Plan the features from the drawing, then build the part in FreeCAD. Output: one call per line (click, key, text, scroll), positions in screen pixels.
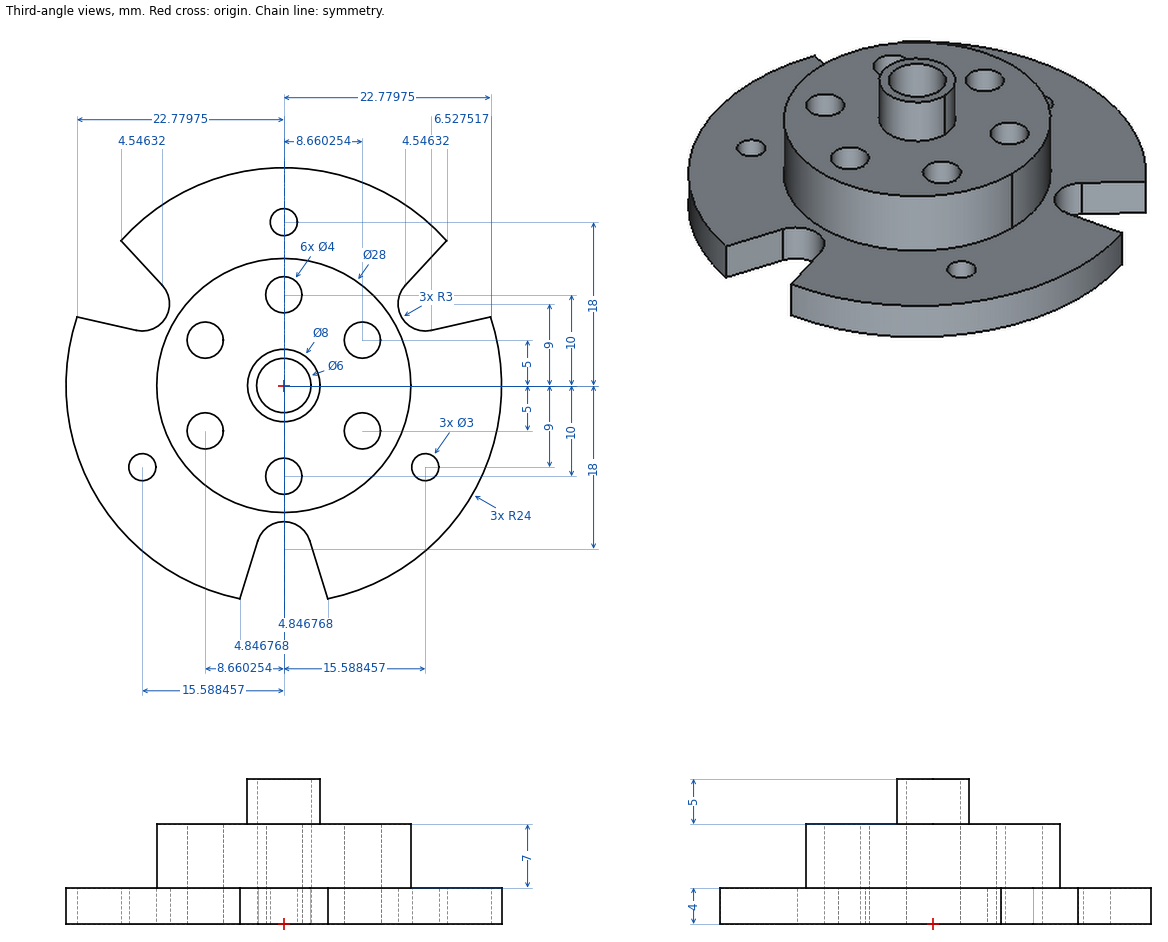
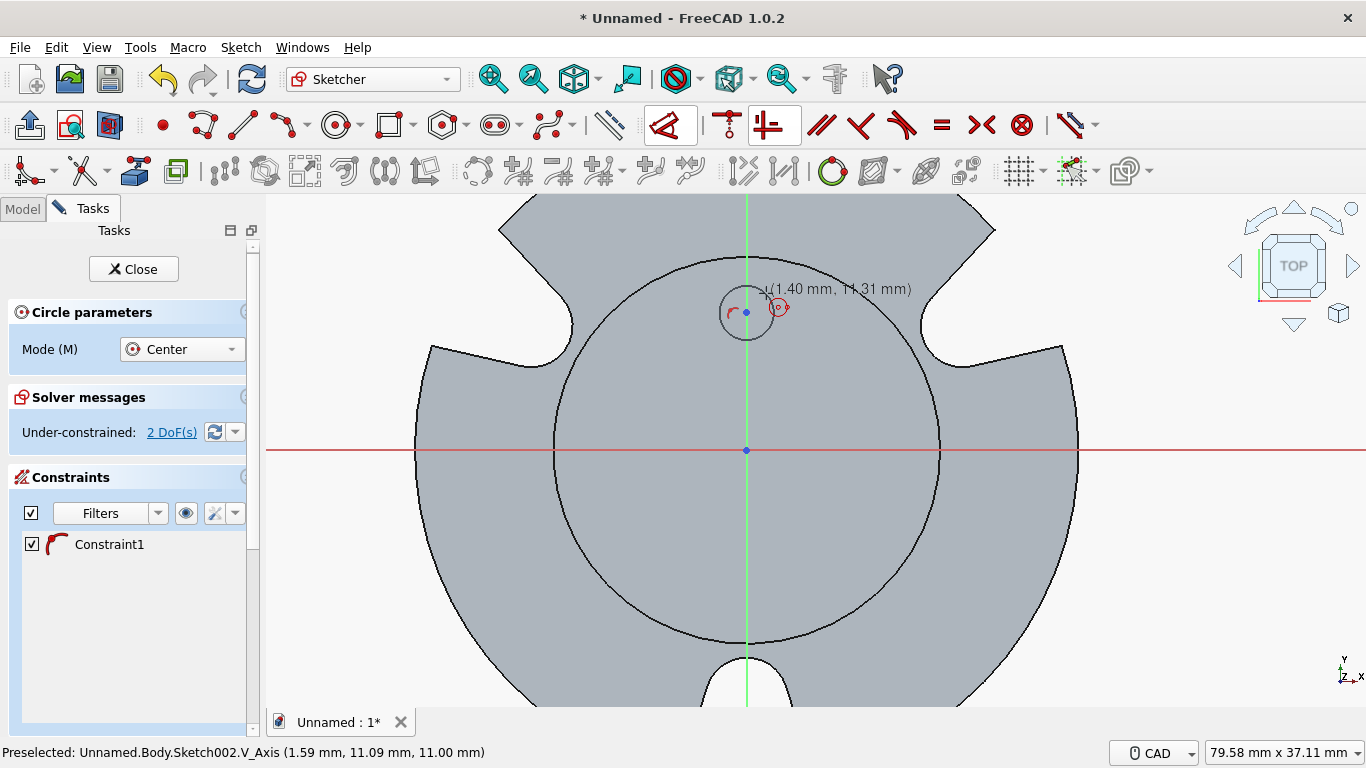
click(866, 381)
click(886, 362)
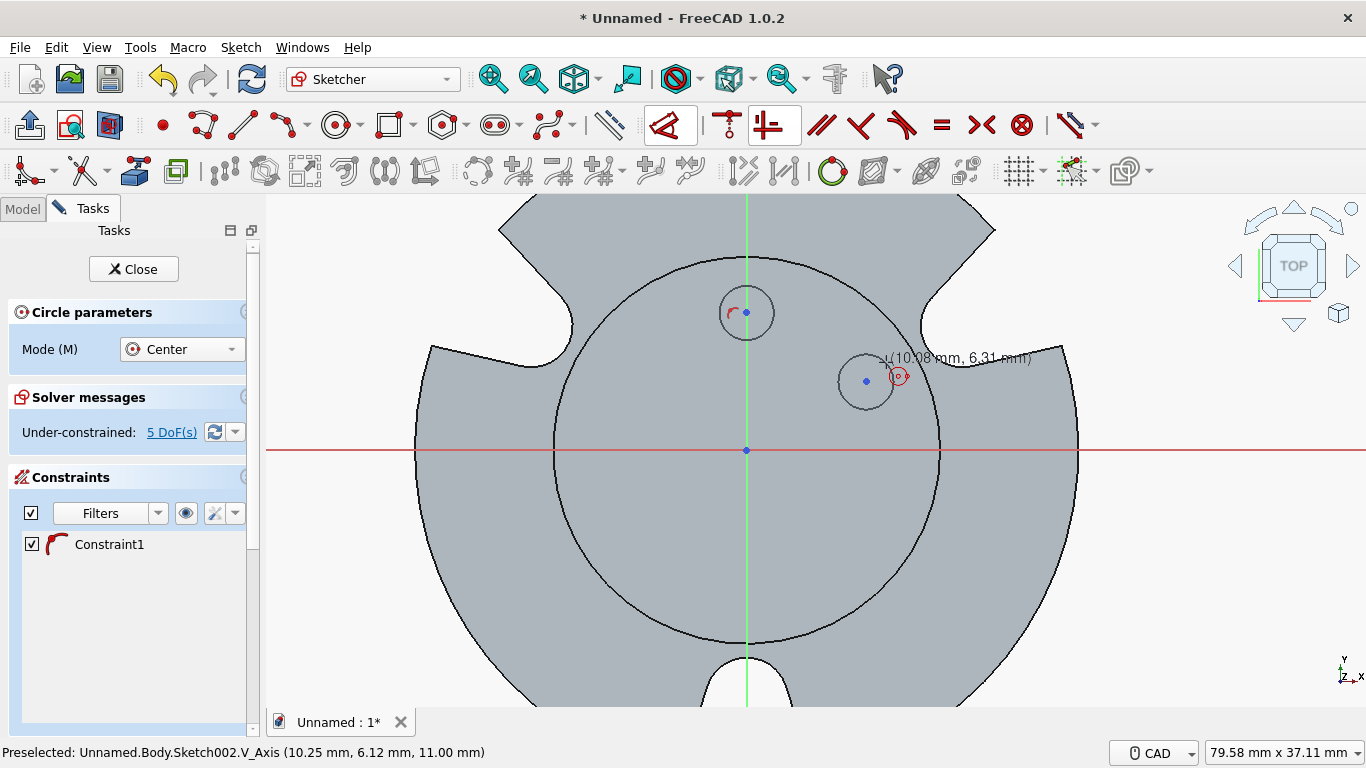
click(866, 519)
click(886, 500)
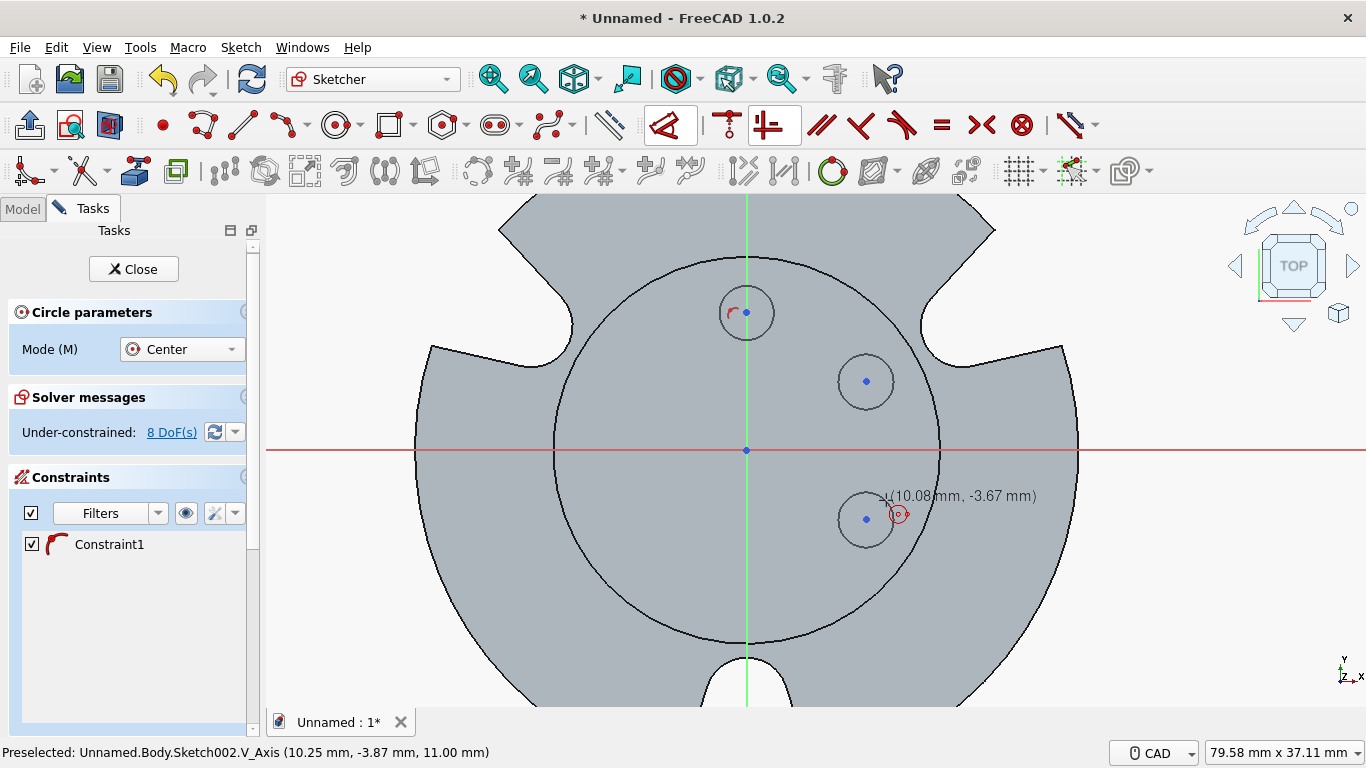
click(747, 589)
click(766, 569)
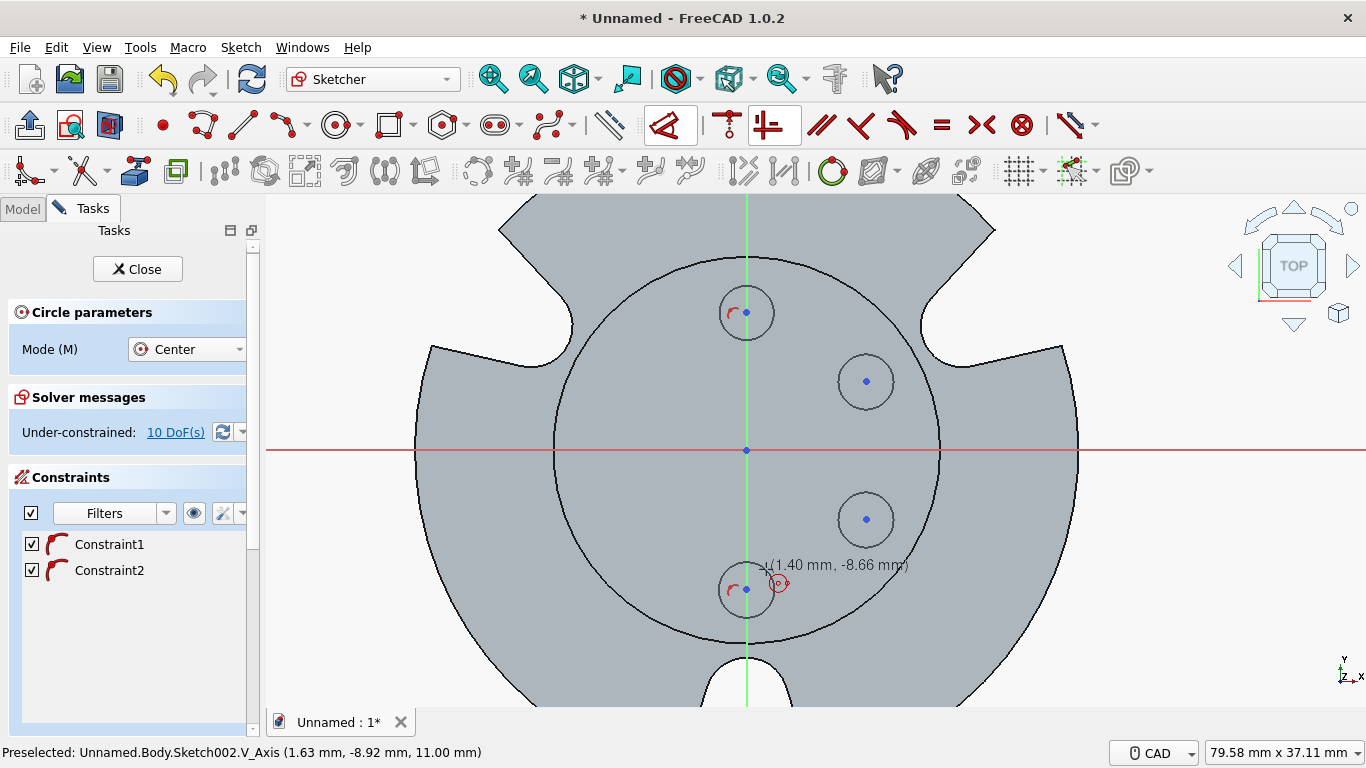
click(627, 519)
click(647, 500)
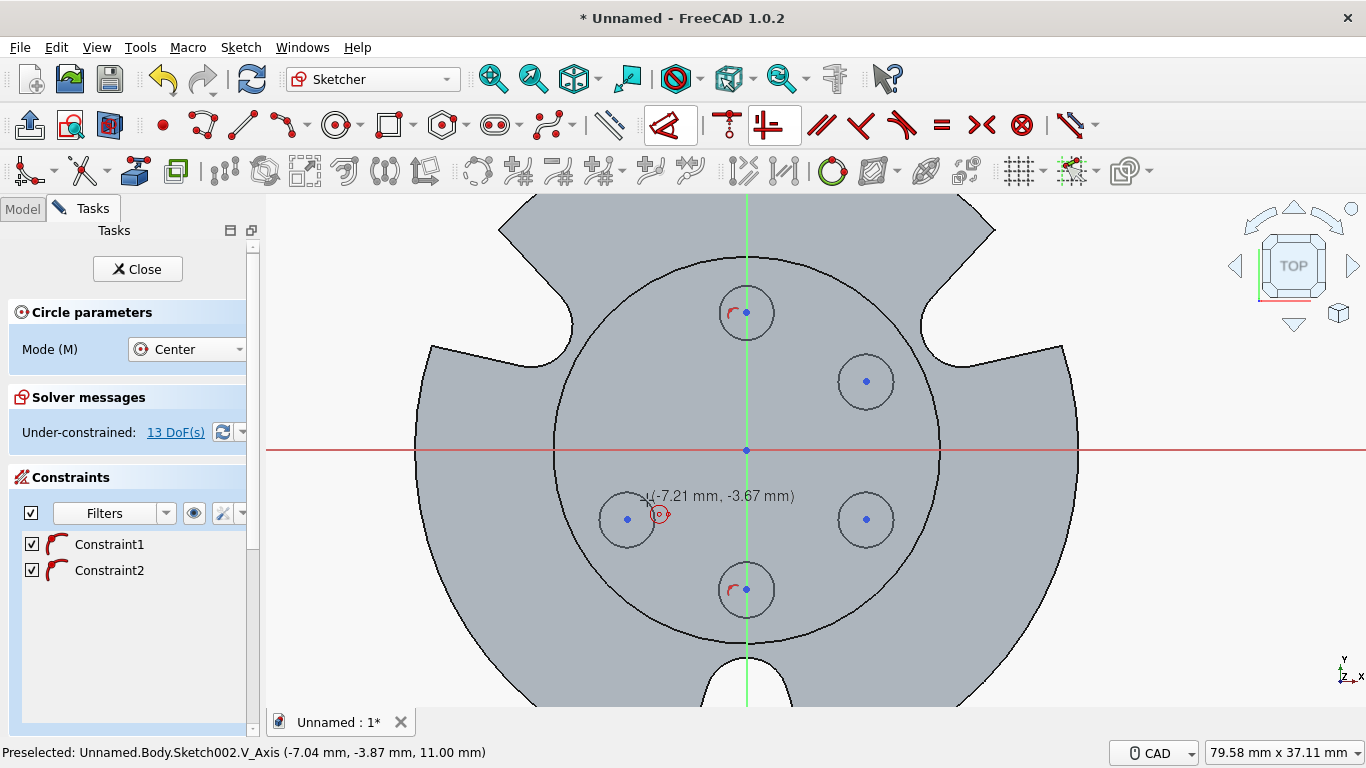
click(627, 381)
click(647, 362)
key(Escape)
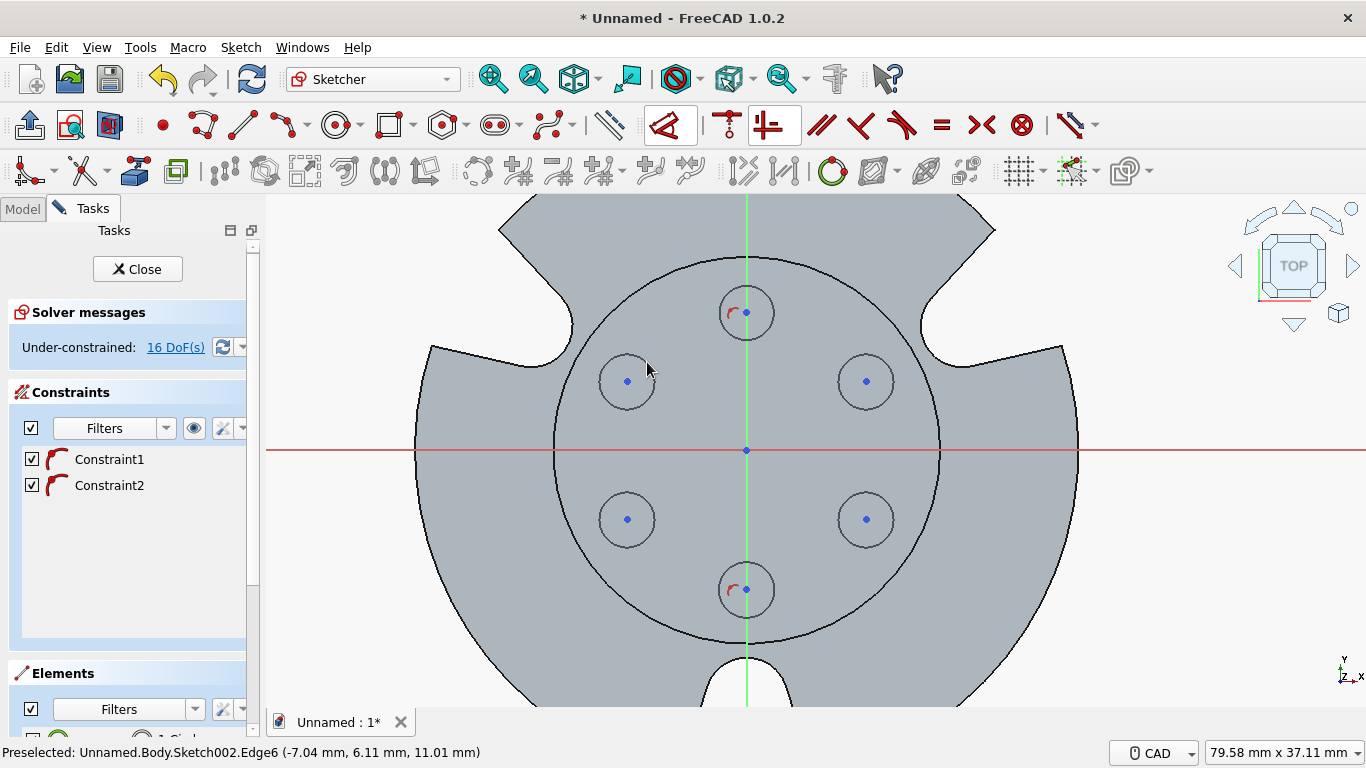
click(766, 294)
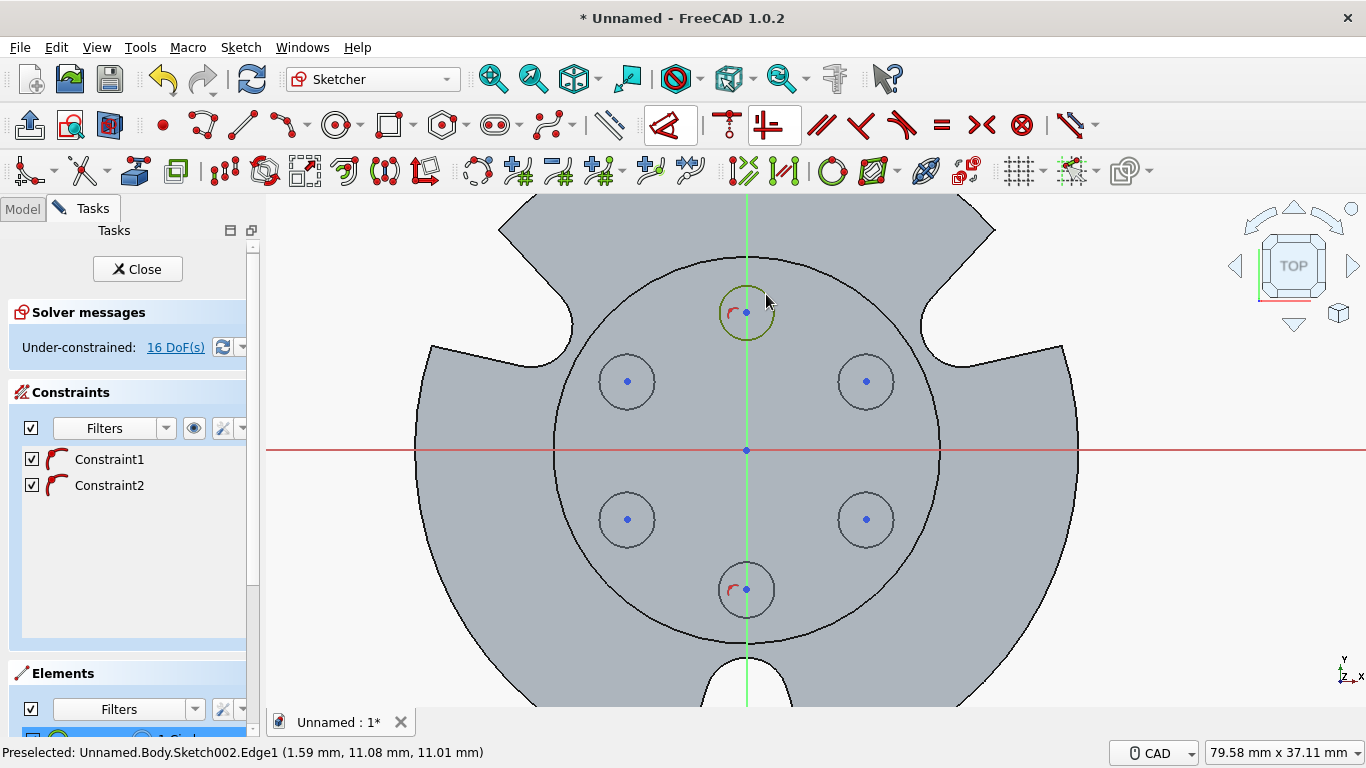
click(885, 362)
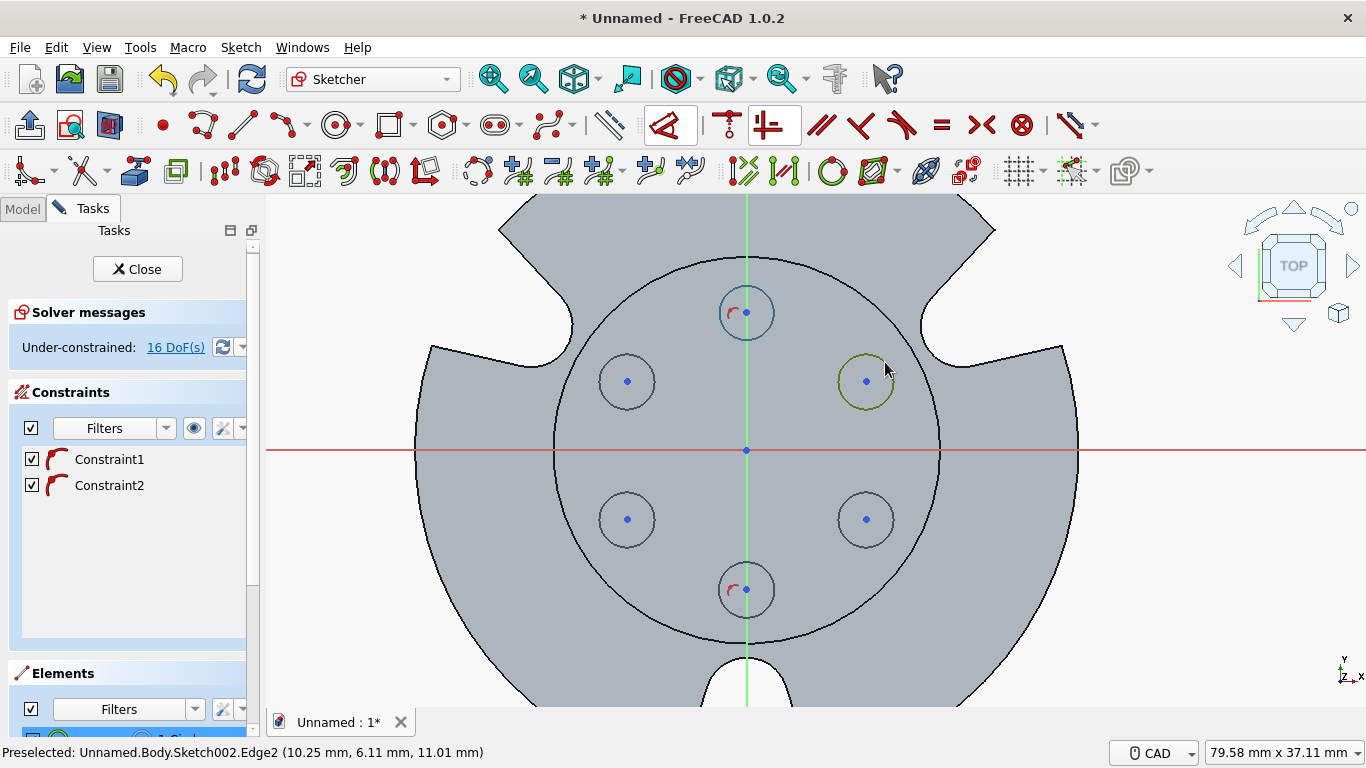
click(885, 500)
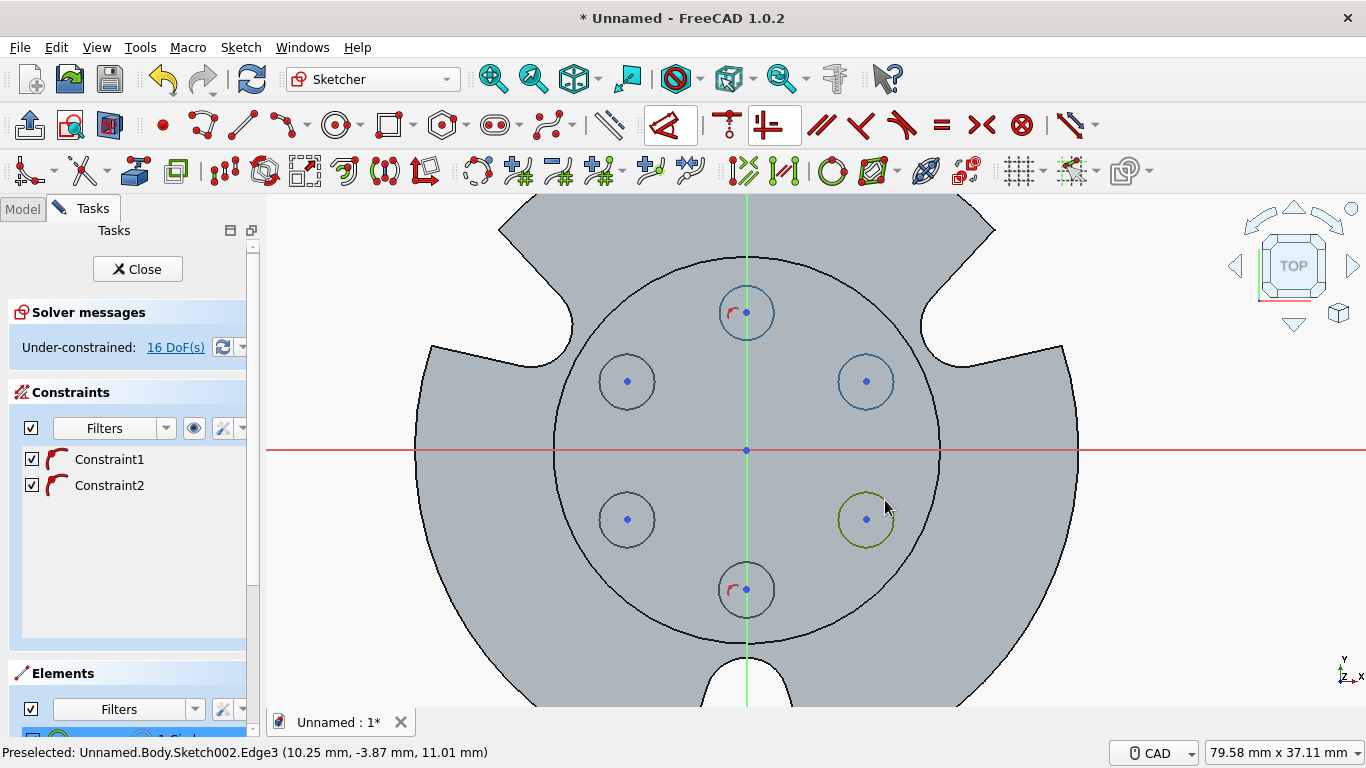
click(766, 570)